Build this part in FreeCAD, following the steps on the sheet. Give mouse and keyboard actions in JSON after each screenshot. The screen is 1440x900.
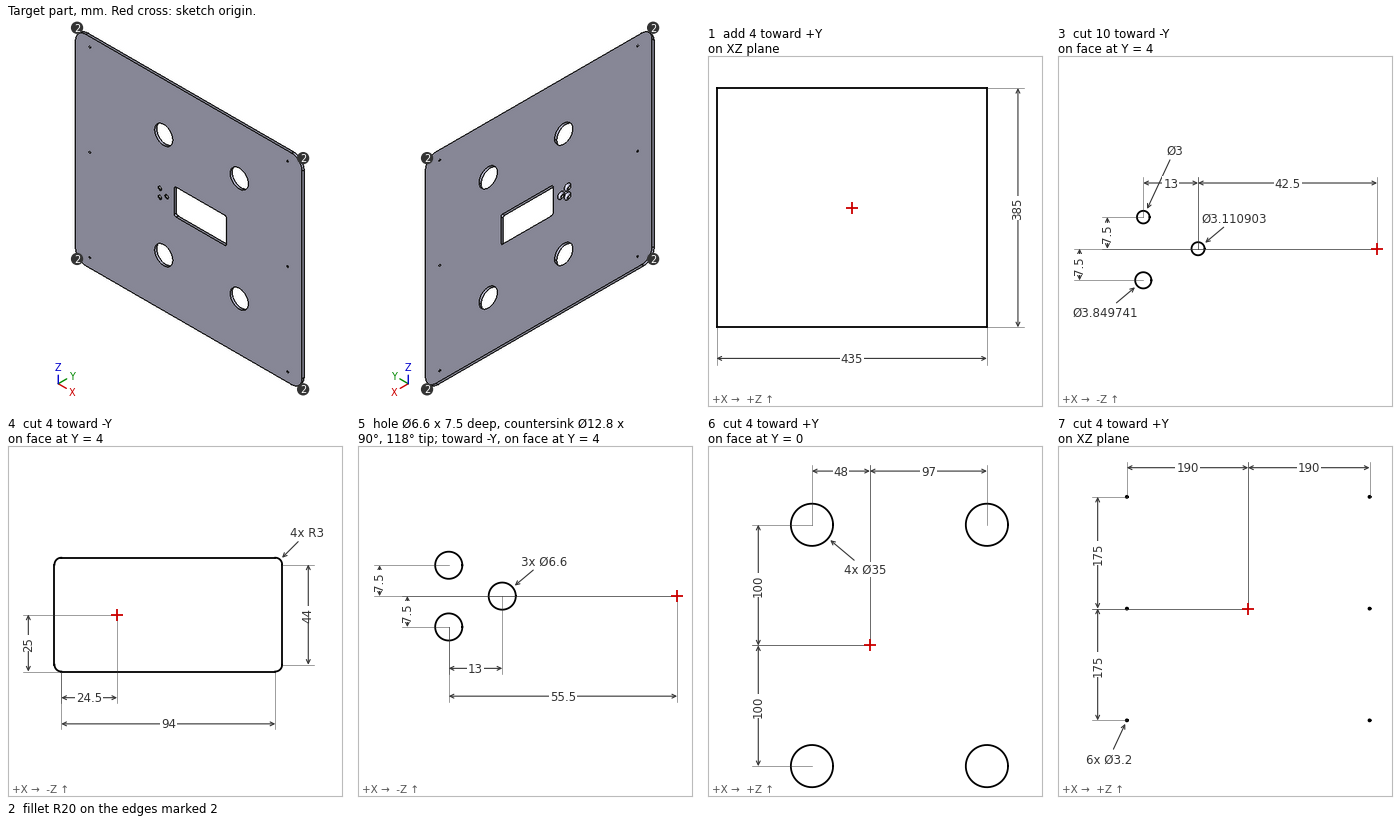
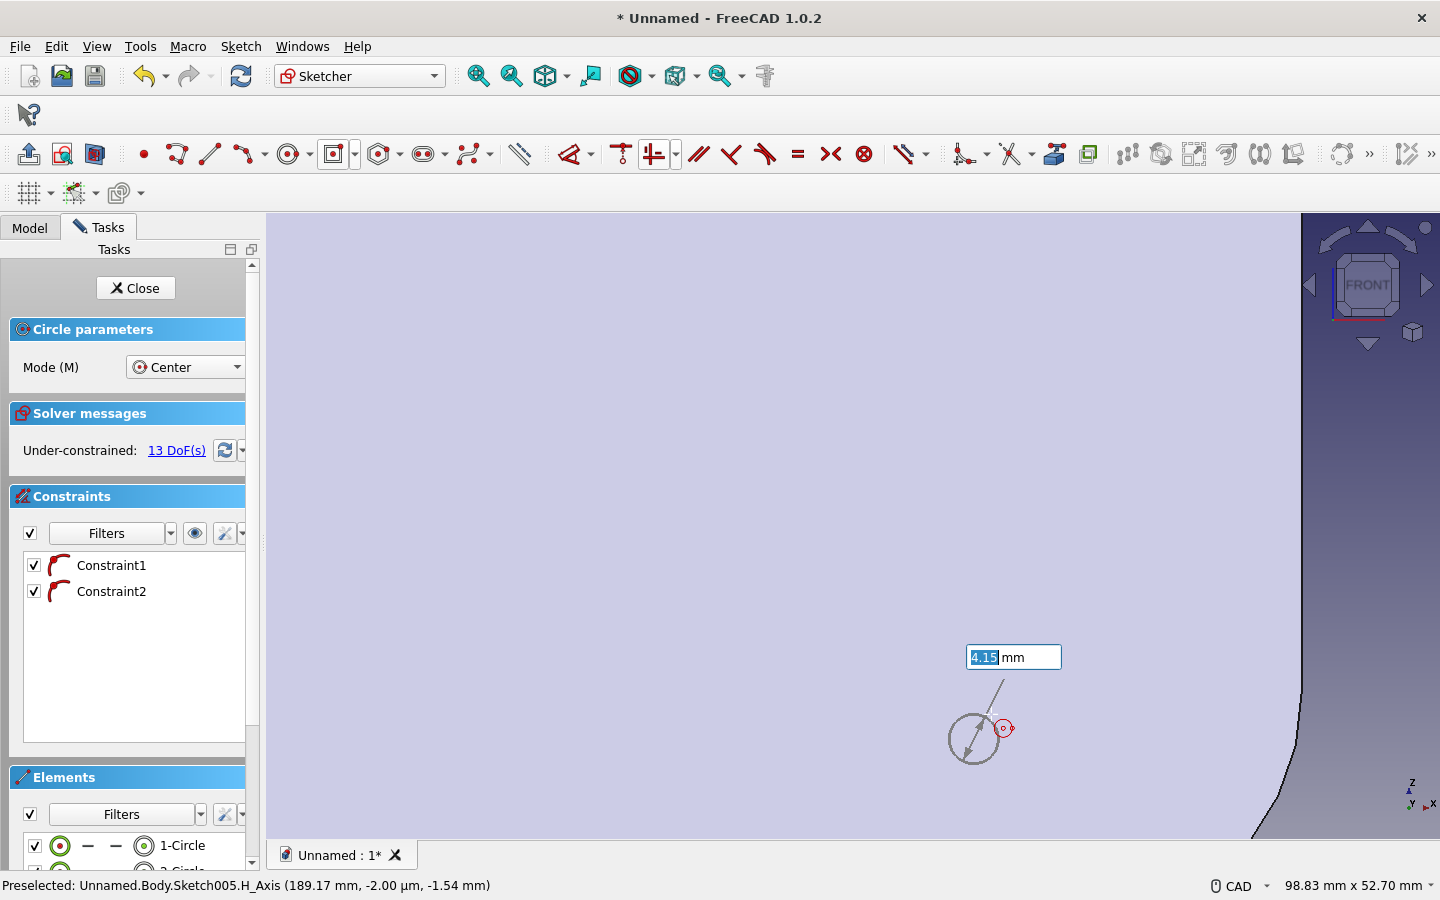
{"action": "left_click", "coordinate": [988, 709]}
{"action": "key", "text": "Escape"}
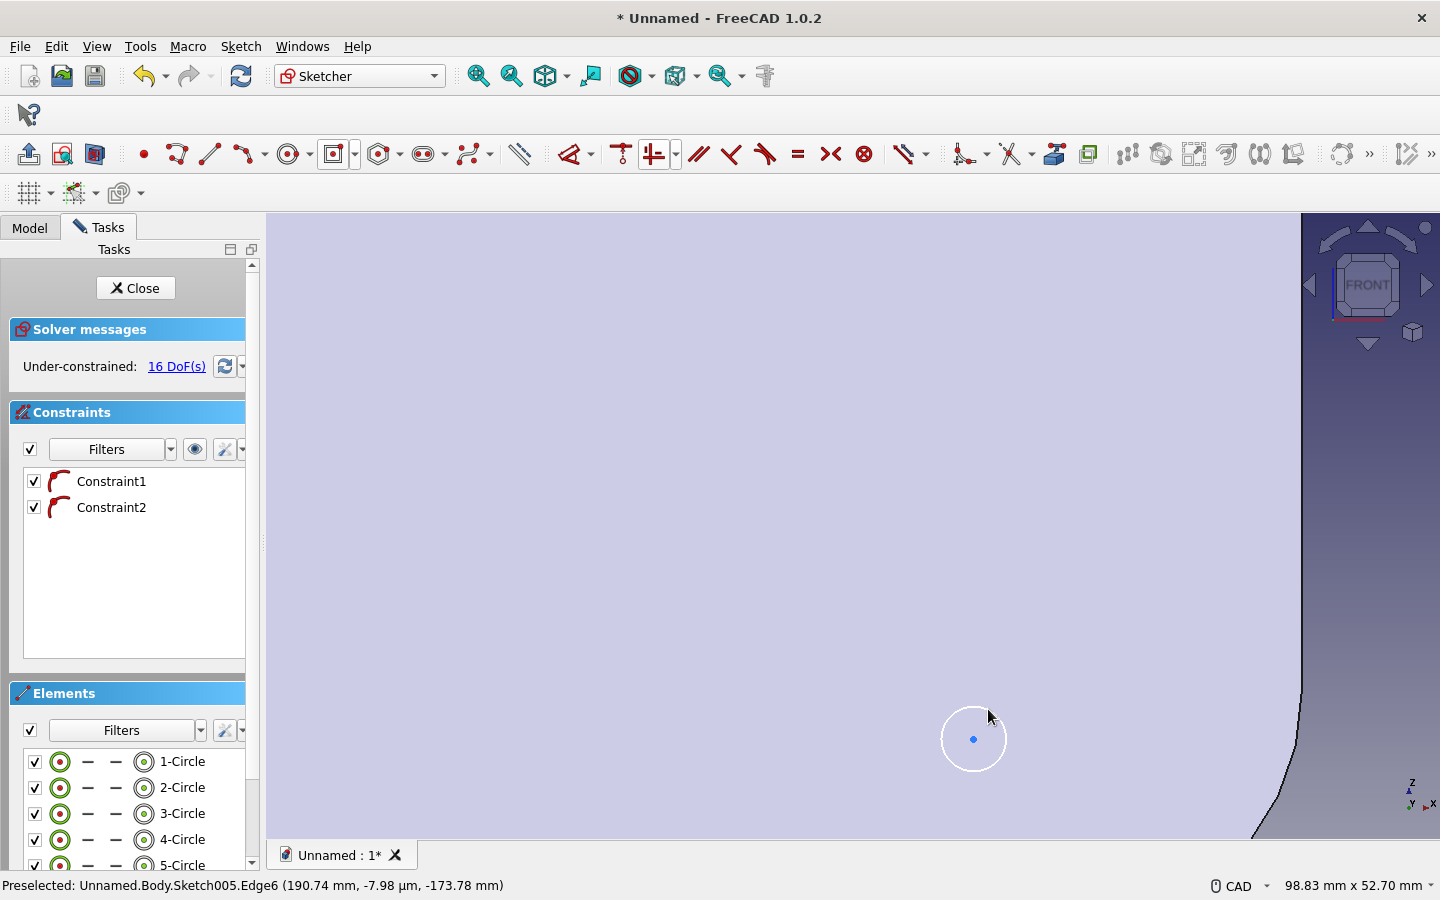
{"action": "scroll", "coordinate": [991, 714], "scroll_direction": "down", "scroll_amount": 12}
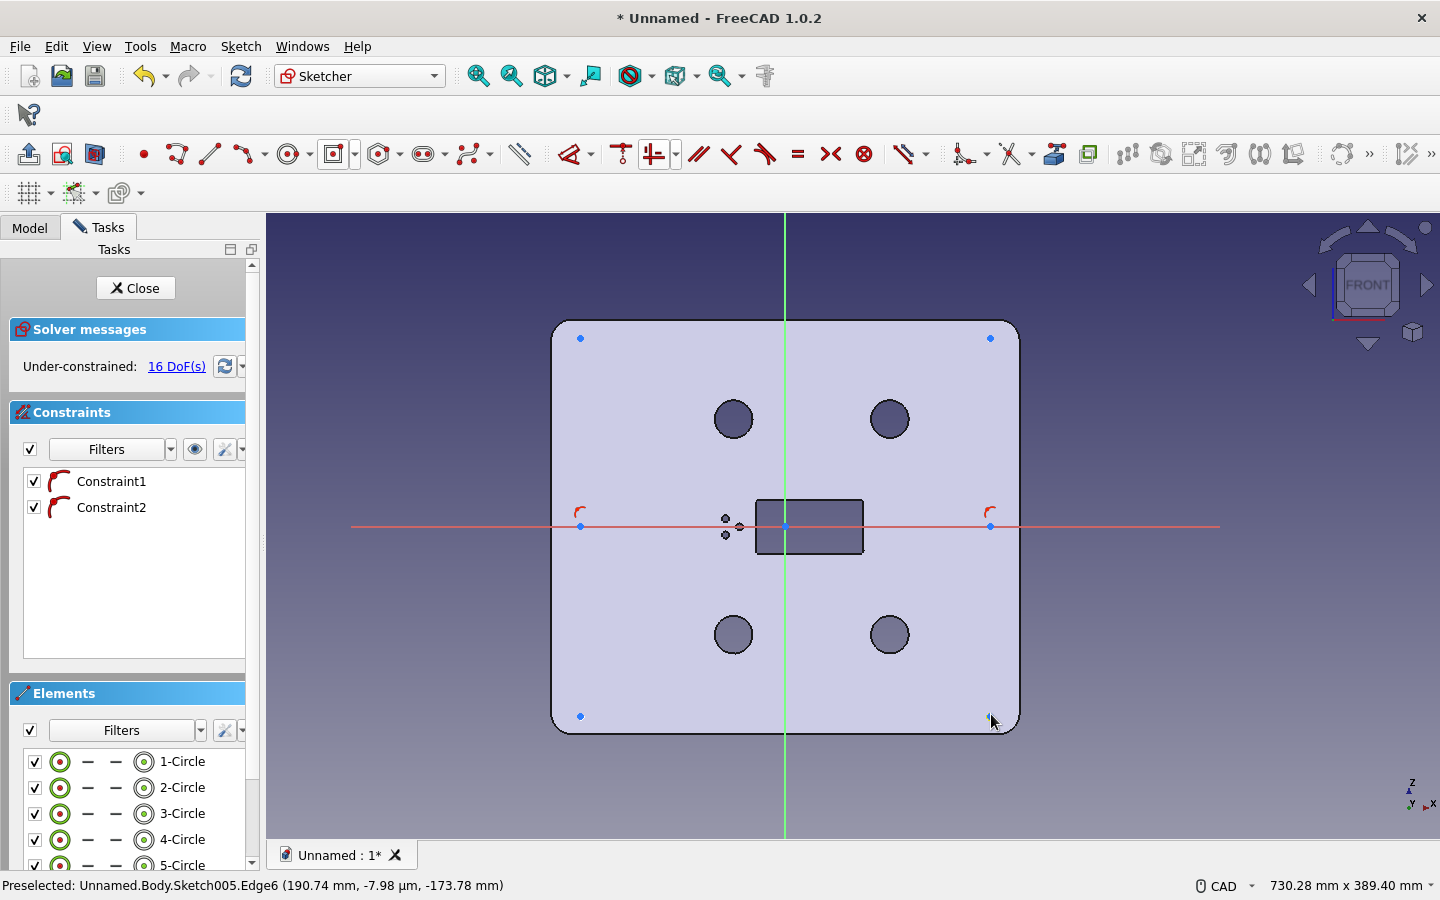
{"action": "scroll", "coordinate": [582, 338], "scroll_direction": "up", "scroll_amount": 10}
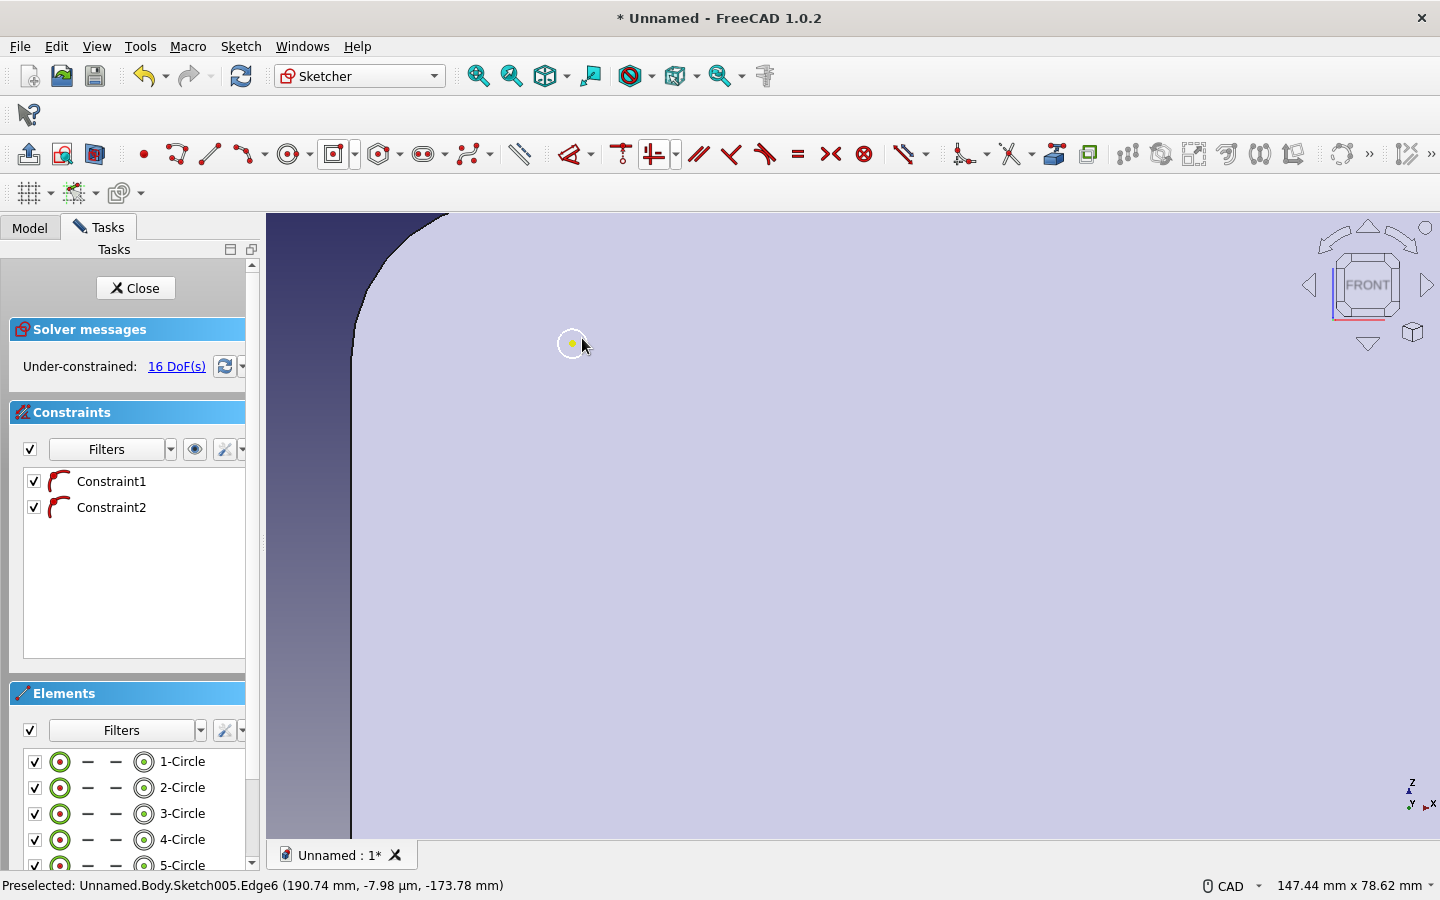
{"action": "left_click", "coordinate": [582, 334]}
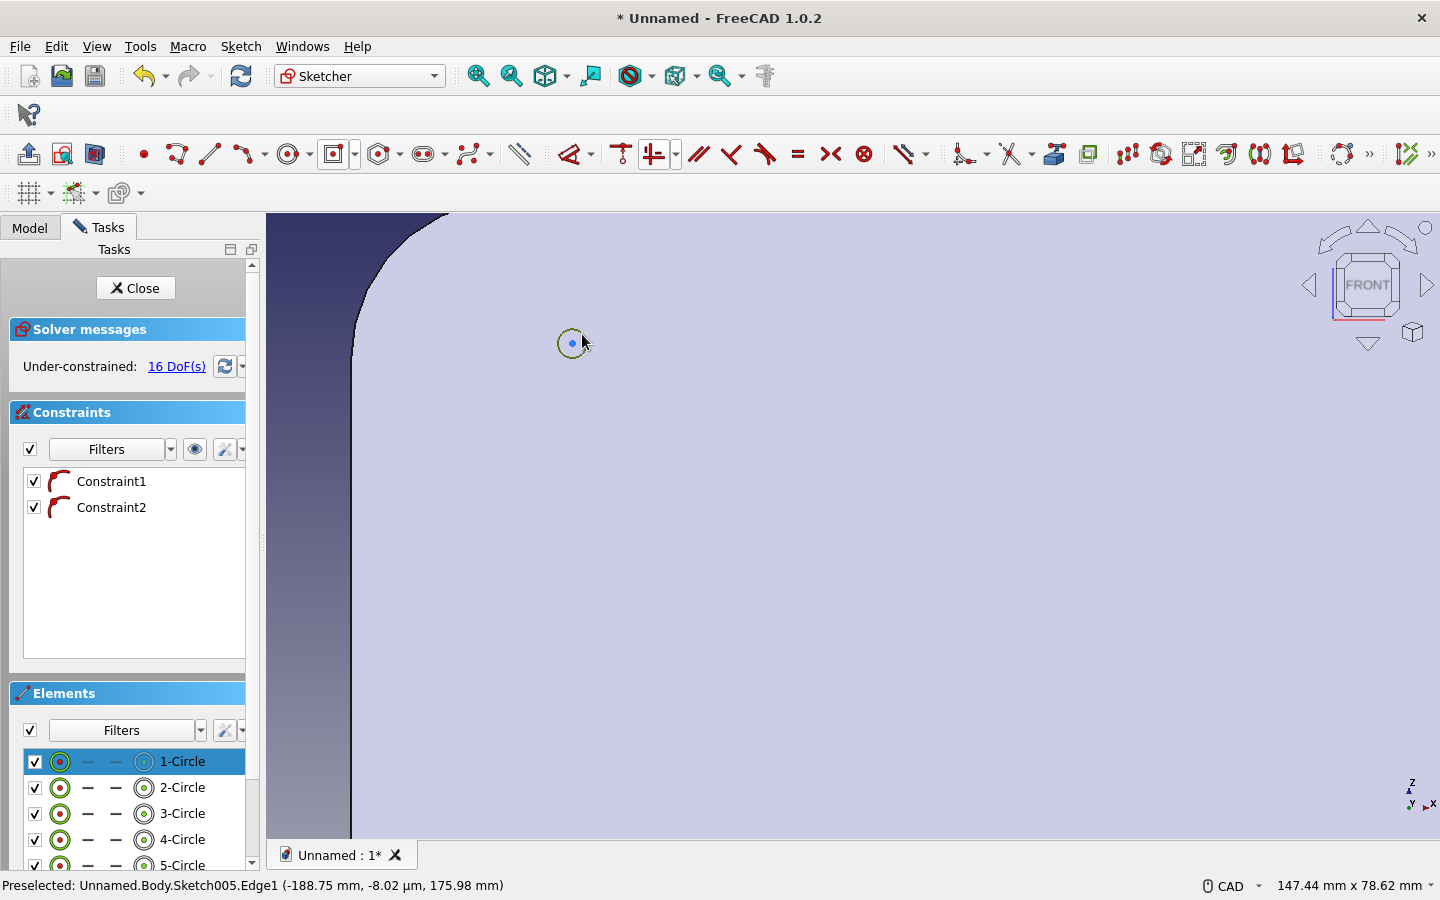
{"action": "scroll", "coordinate": [581, 337], "scroll_direction": "down", "scroll_amount": 10}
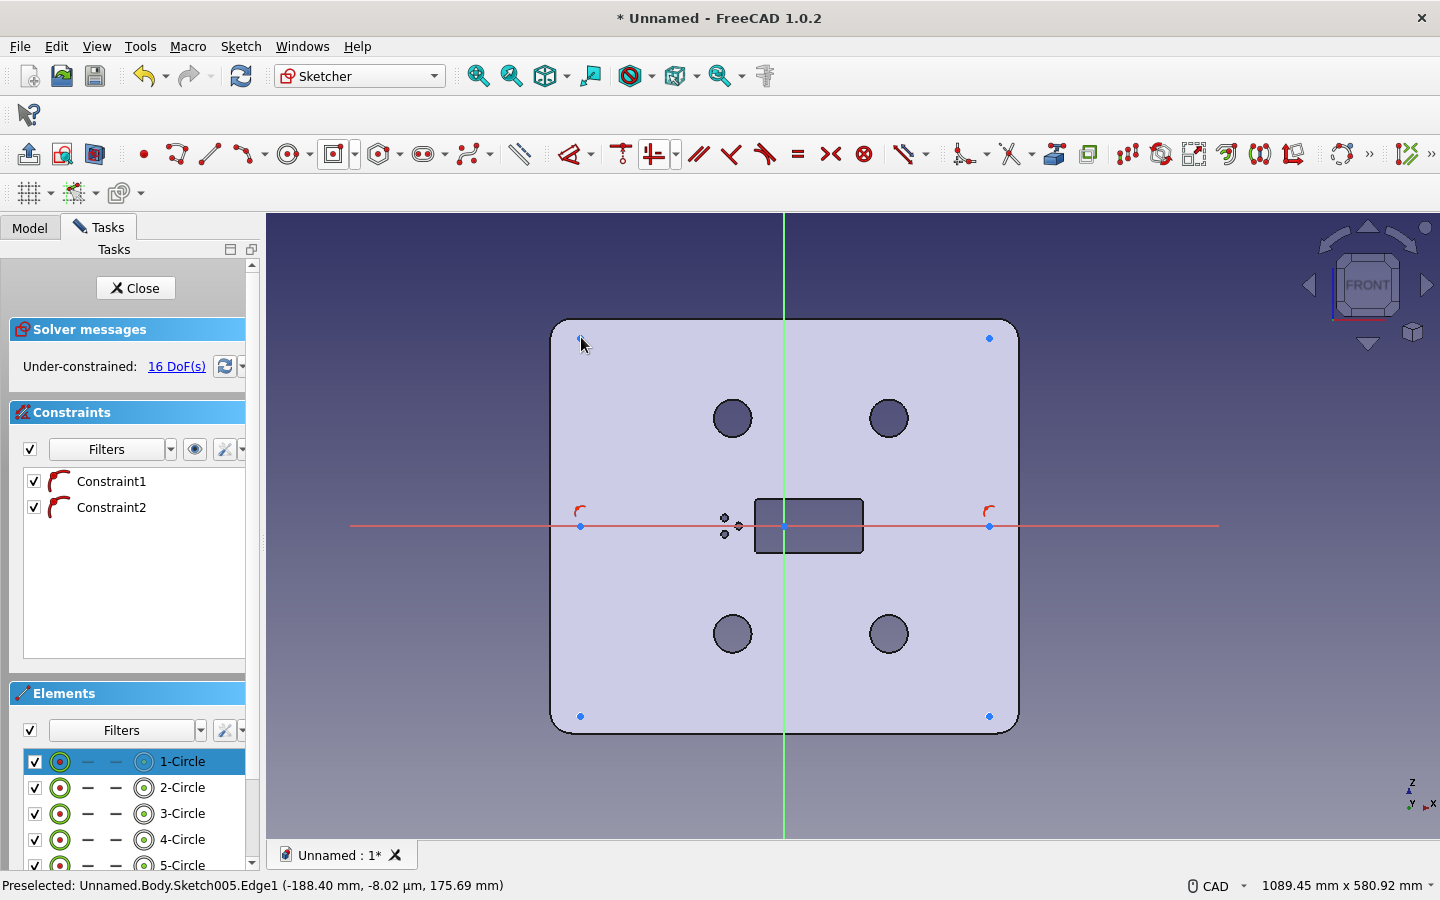
{"action": "scroll", "coordinate": [581, 525], "scroll_direction": "up", "scroll_amount": 12}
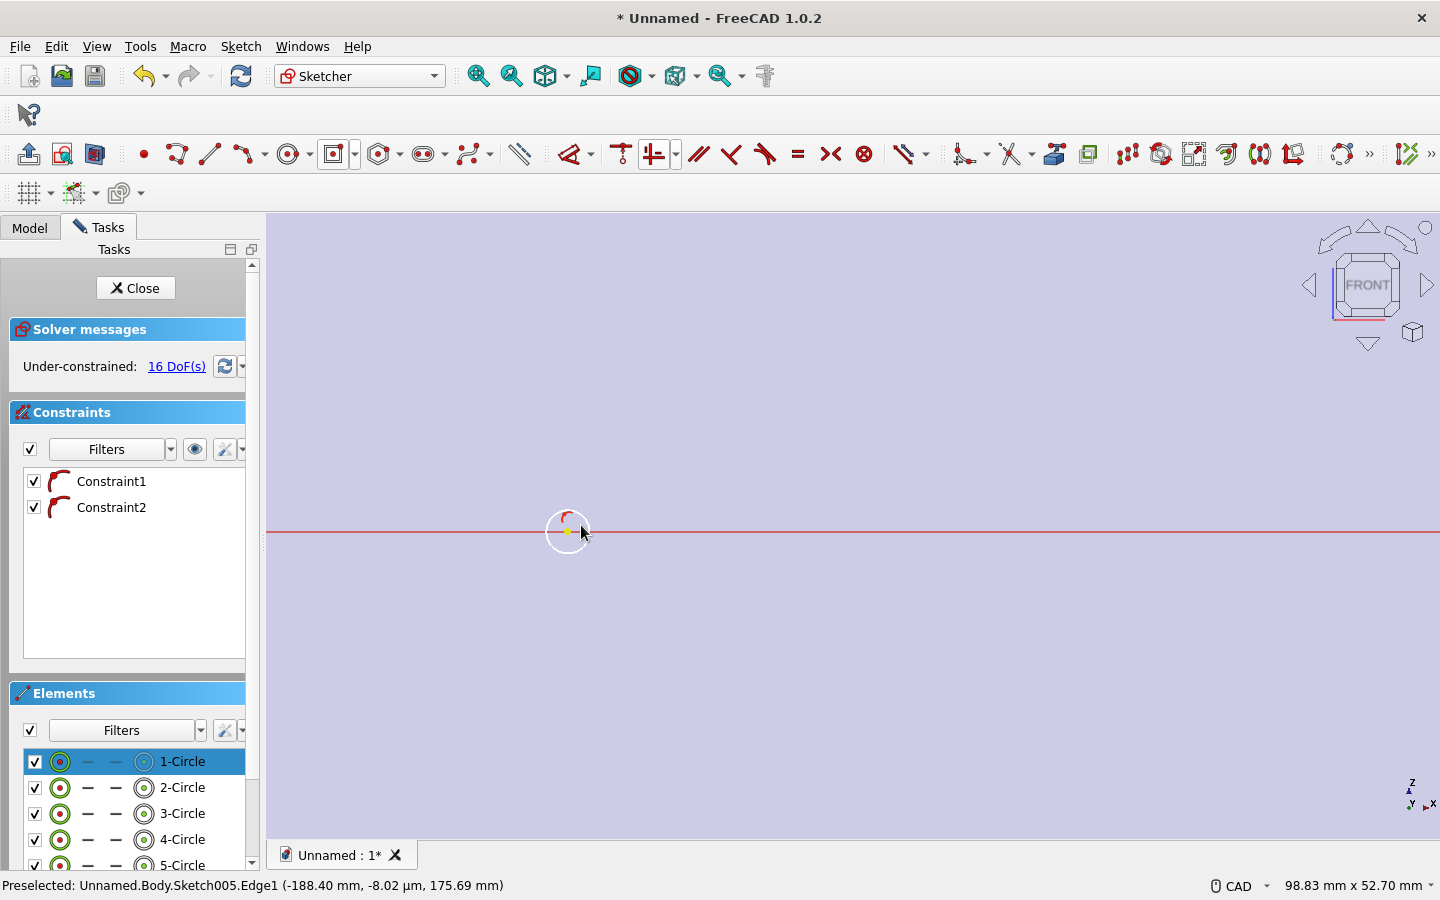
{"action": "left_click", "coordinate": [583, 517]}